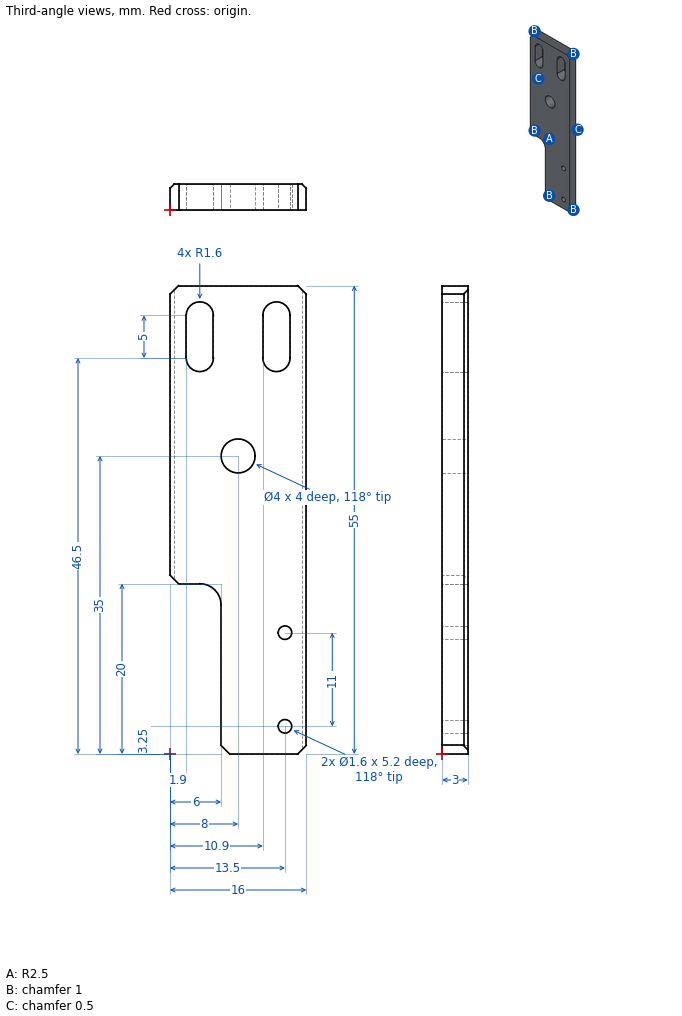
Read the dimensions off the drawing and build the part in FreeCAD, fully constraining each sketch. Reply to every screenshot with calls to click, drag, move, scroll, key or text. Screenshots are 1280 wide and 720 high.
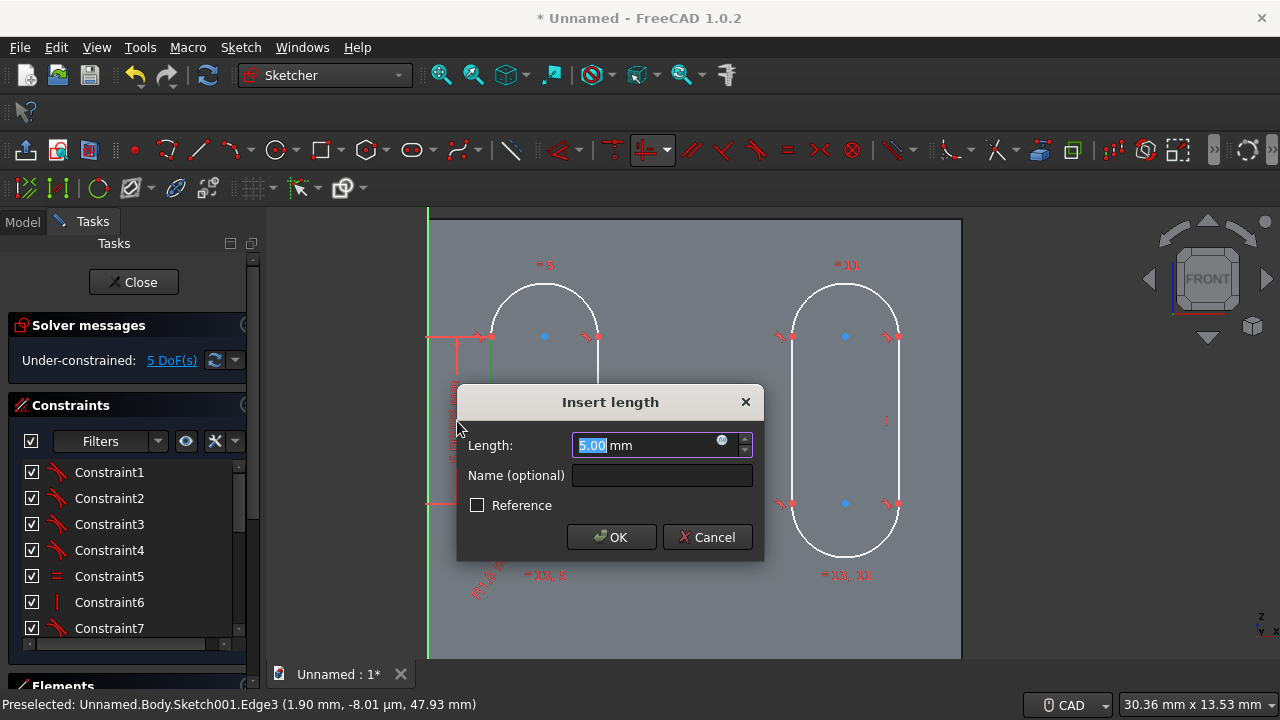
text(5)
key(Return)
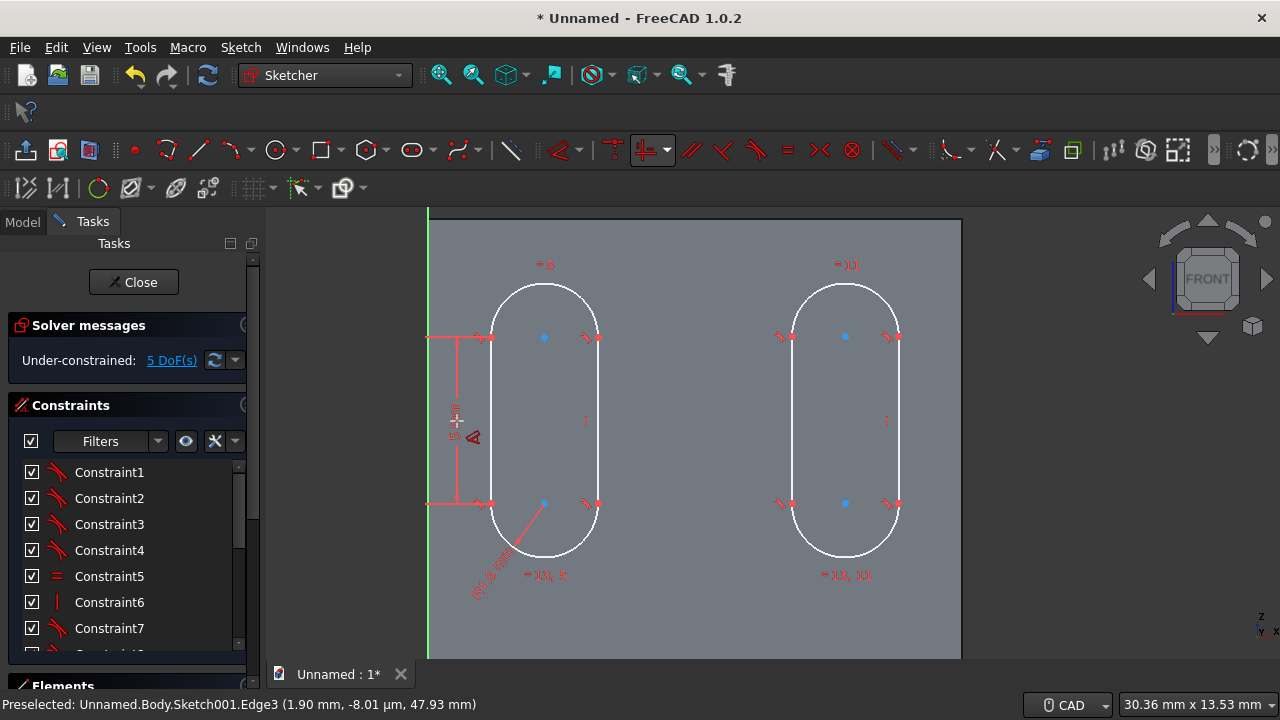
click(792, 454)
click(826, 421)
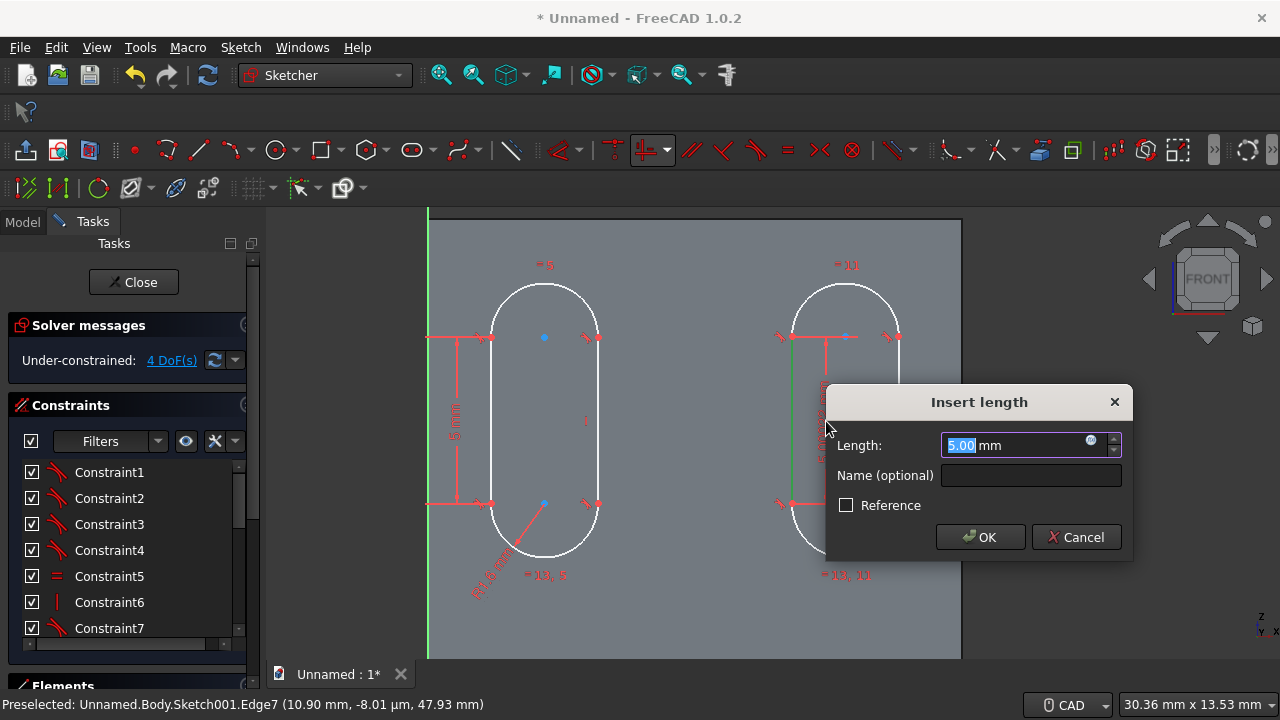
text(5)
key(Return)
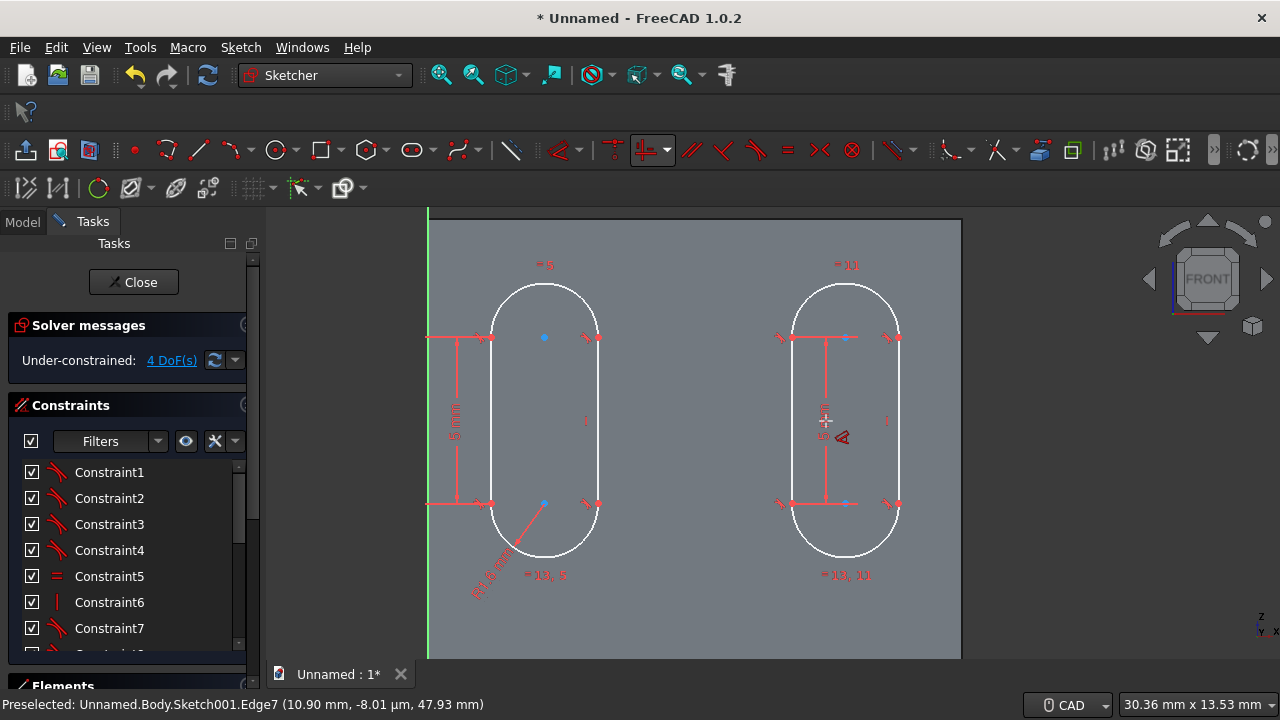
click(491, 504)
click(459, 470)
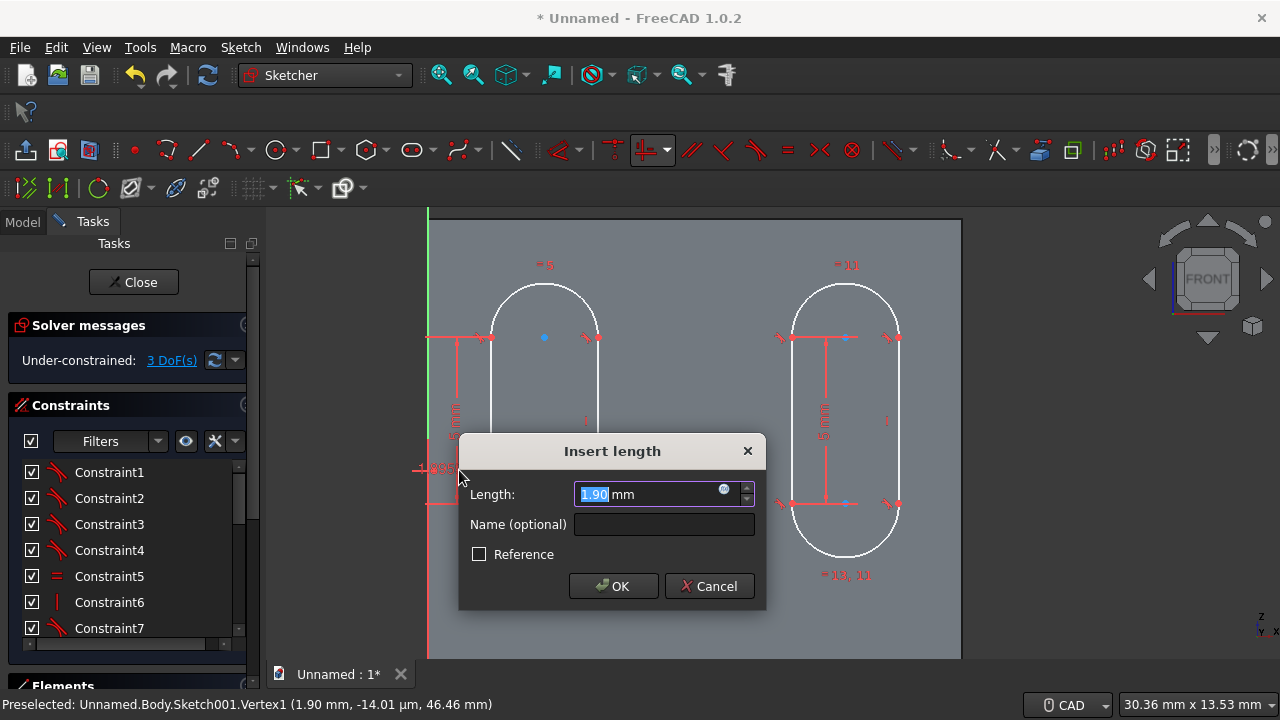
text(1.9)
key(Return)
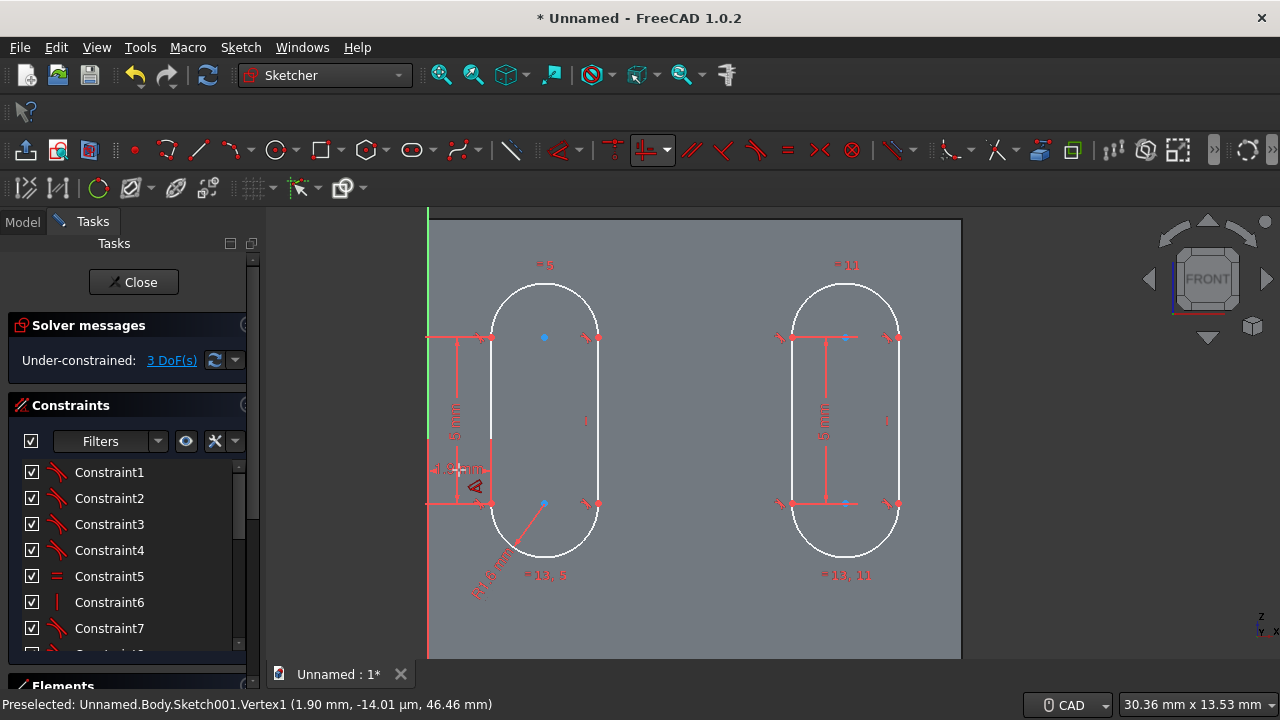
click(491, 504)
click(394, 568)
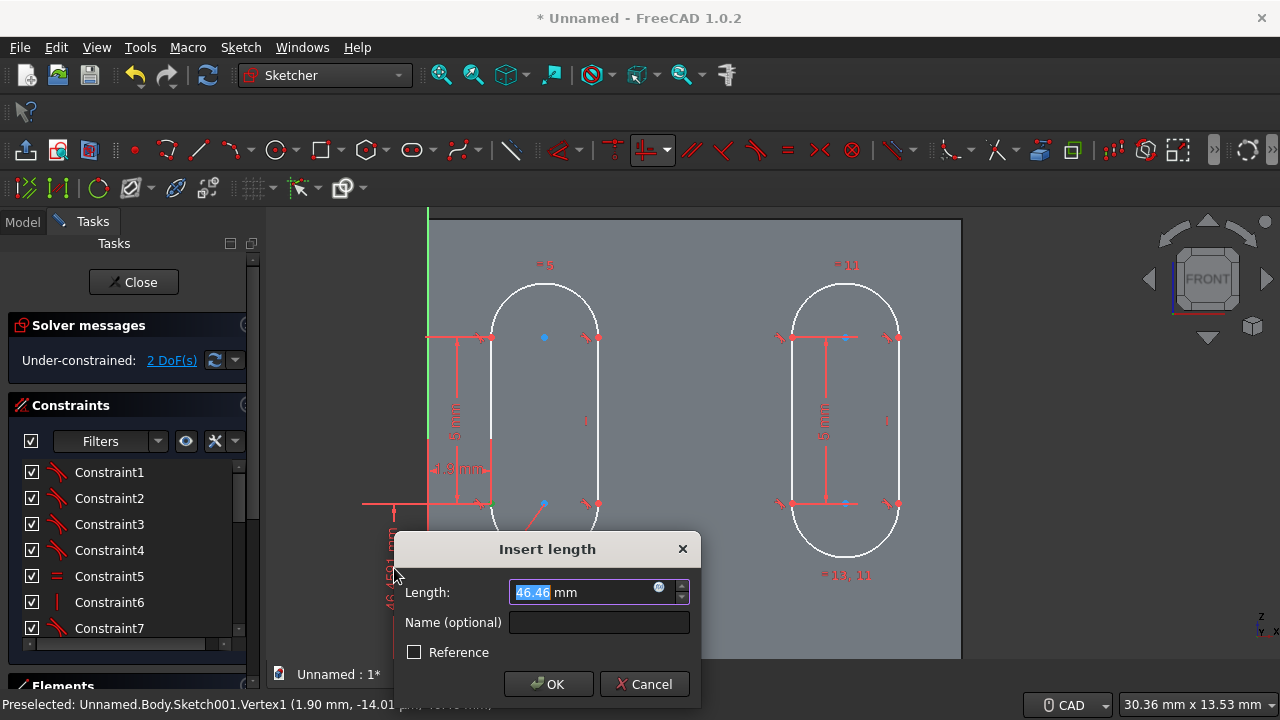
text(46.5)
key(Return)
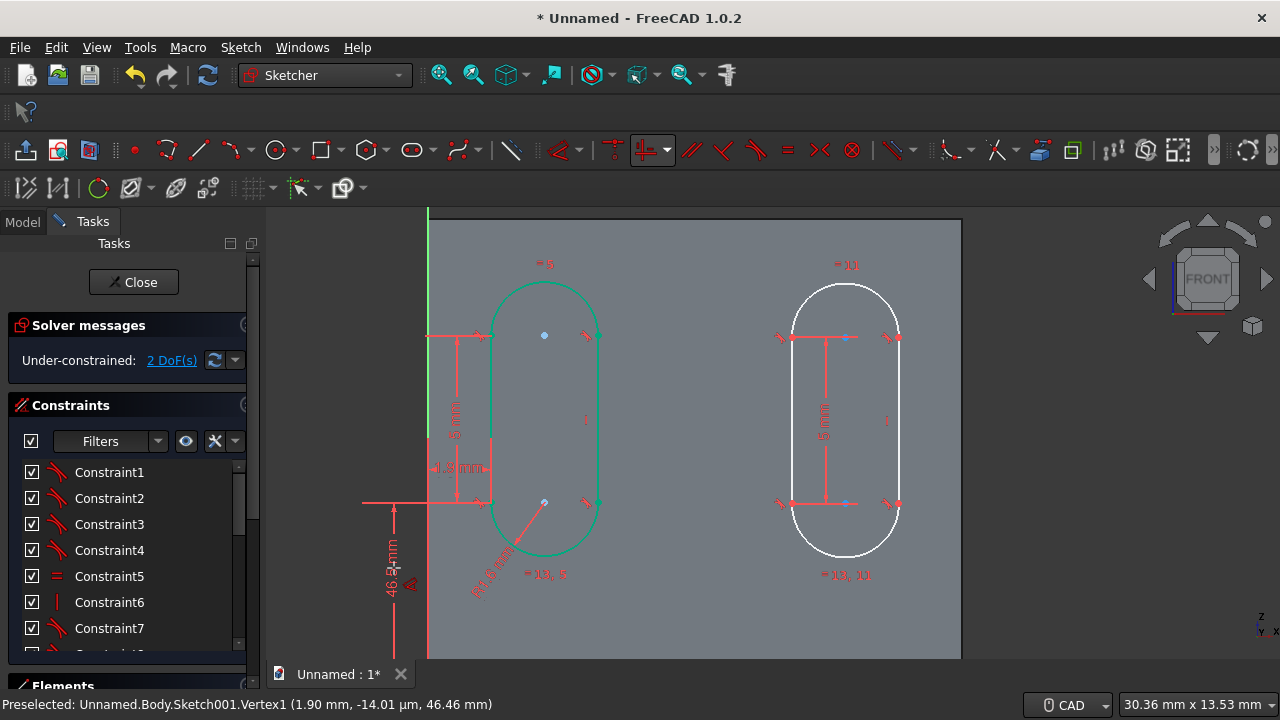
click(792, 504)
click(694, 470)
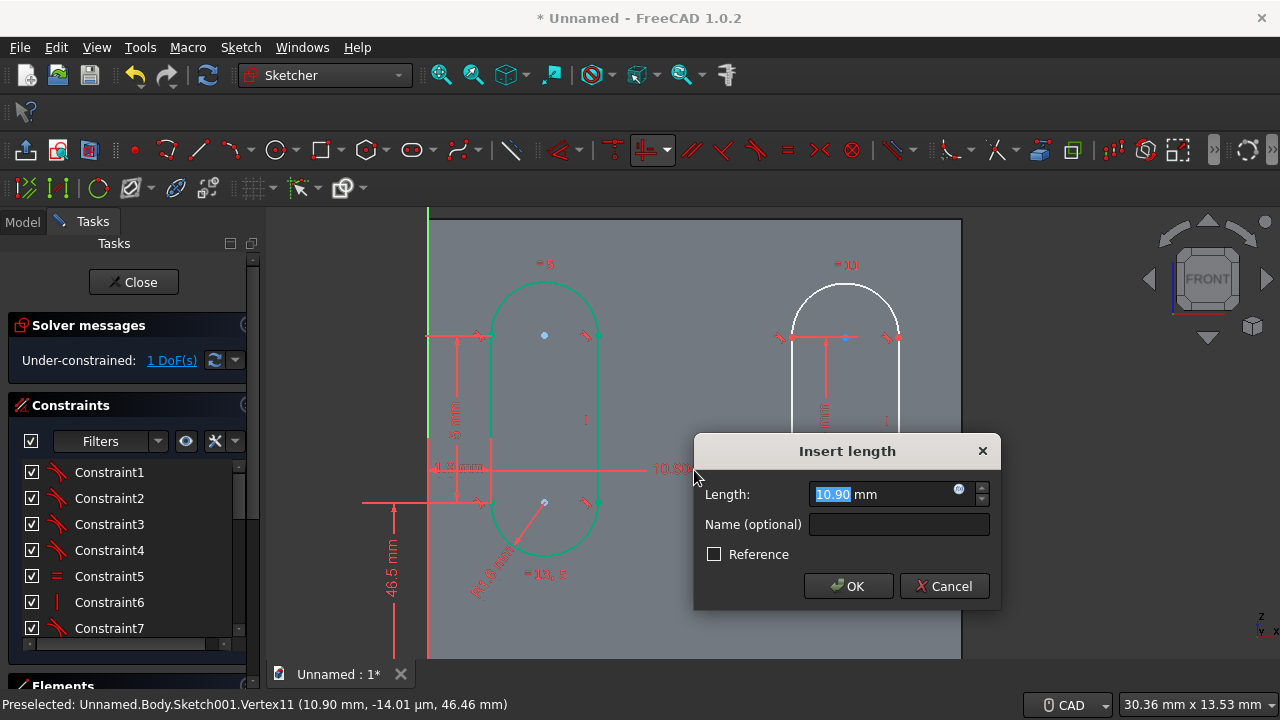
text(10.9)
key(Return)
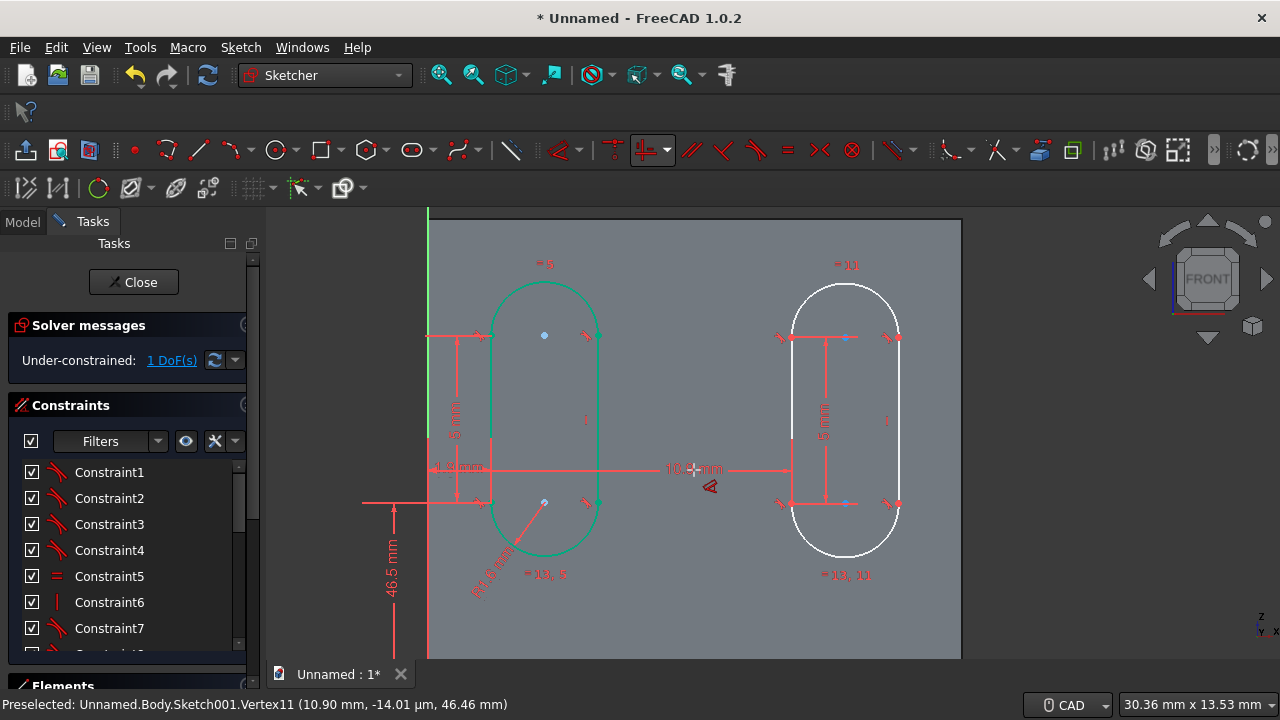
click(792, 504)
click(394, 538)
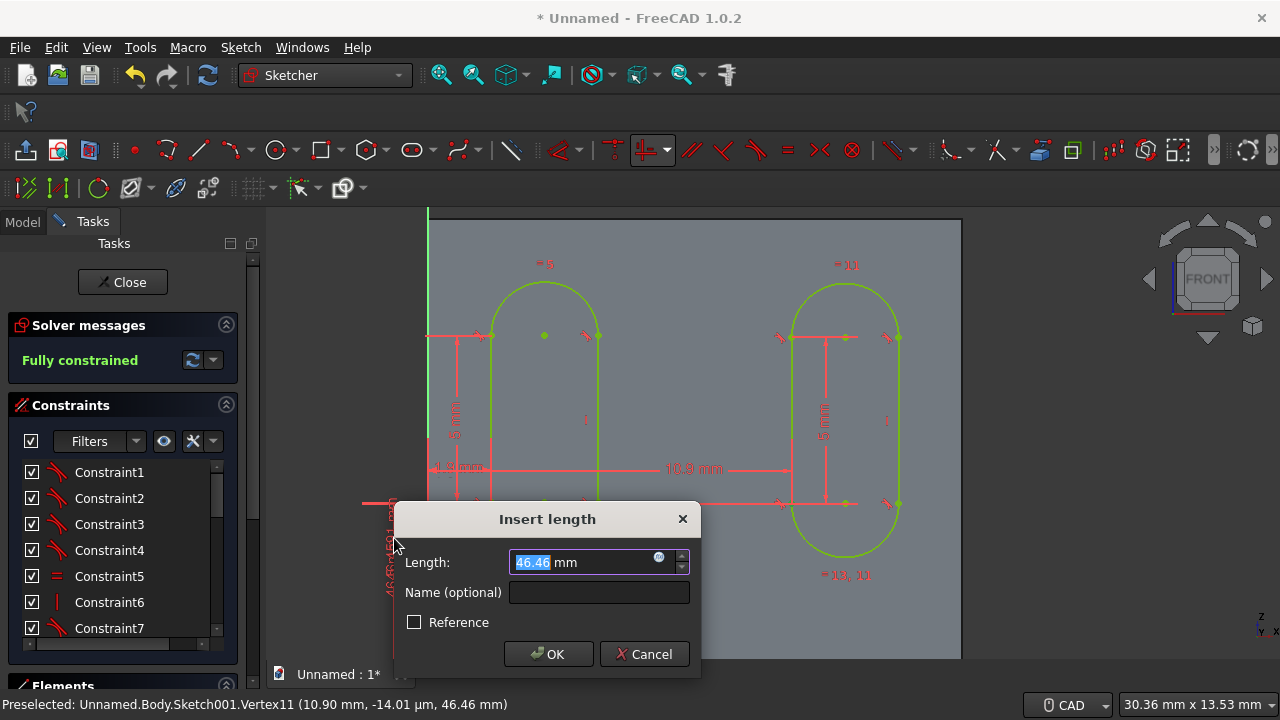
text(46.5)
key(Return)
key(Escape)